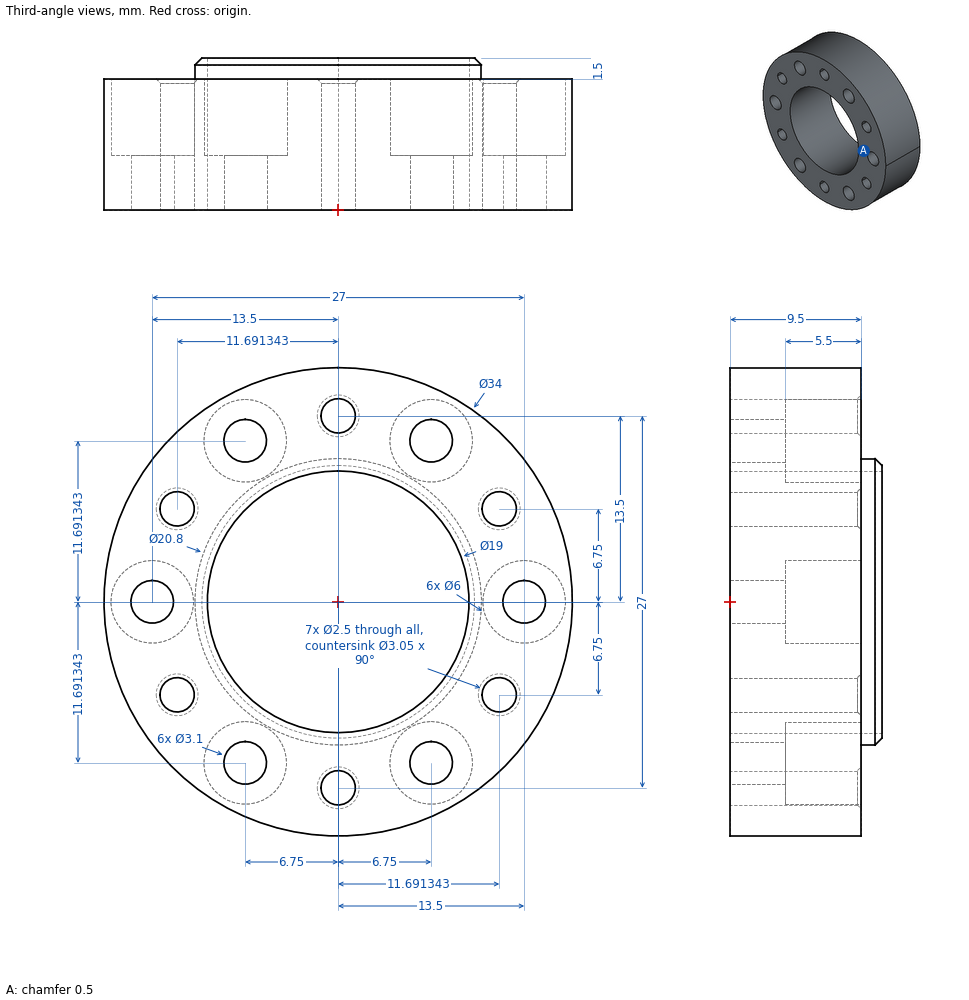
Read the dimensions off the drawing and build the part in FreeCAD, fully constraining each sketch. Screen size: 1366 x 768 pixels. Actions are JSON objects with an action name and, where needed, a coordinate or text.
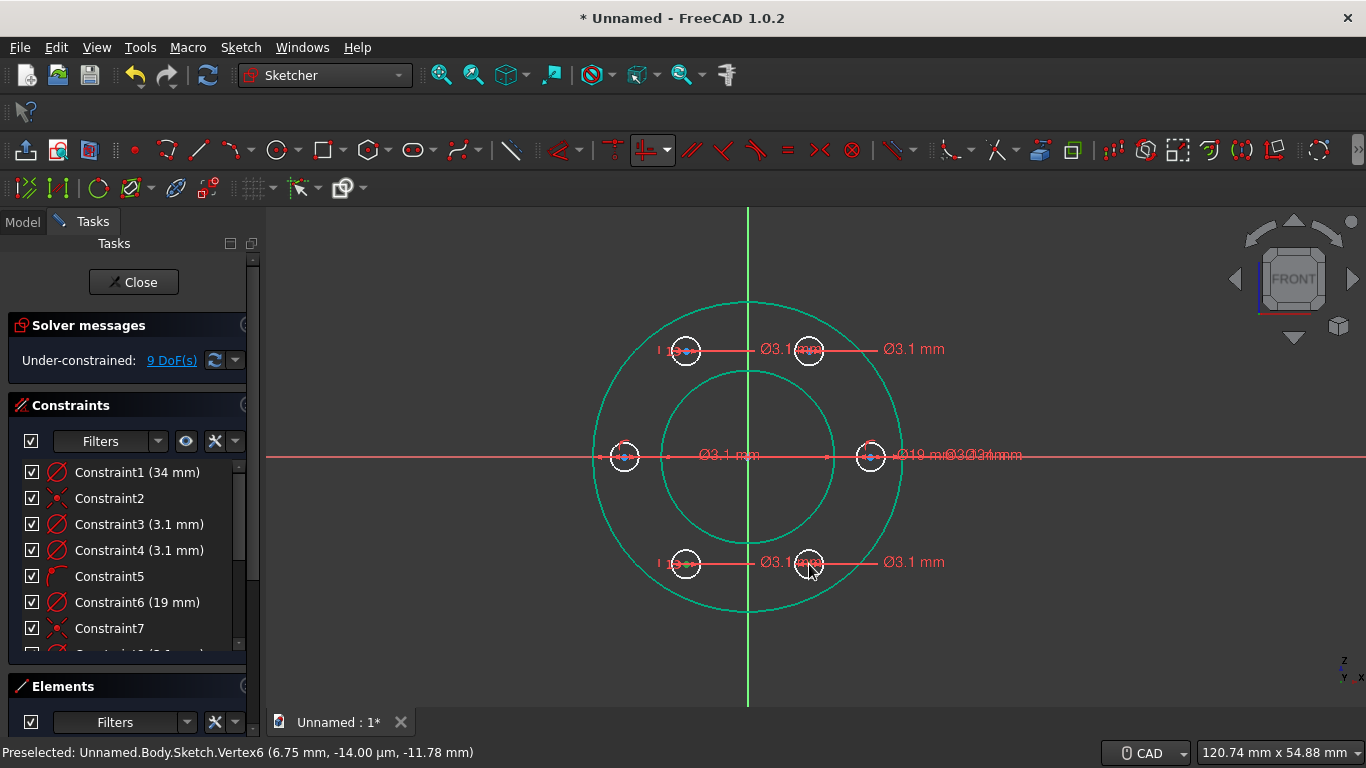
{"action": "left_click", "coordinate": [670, 150]}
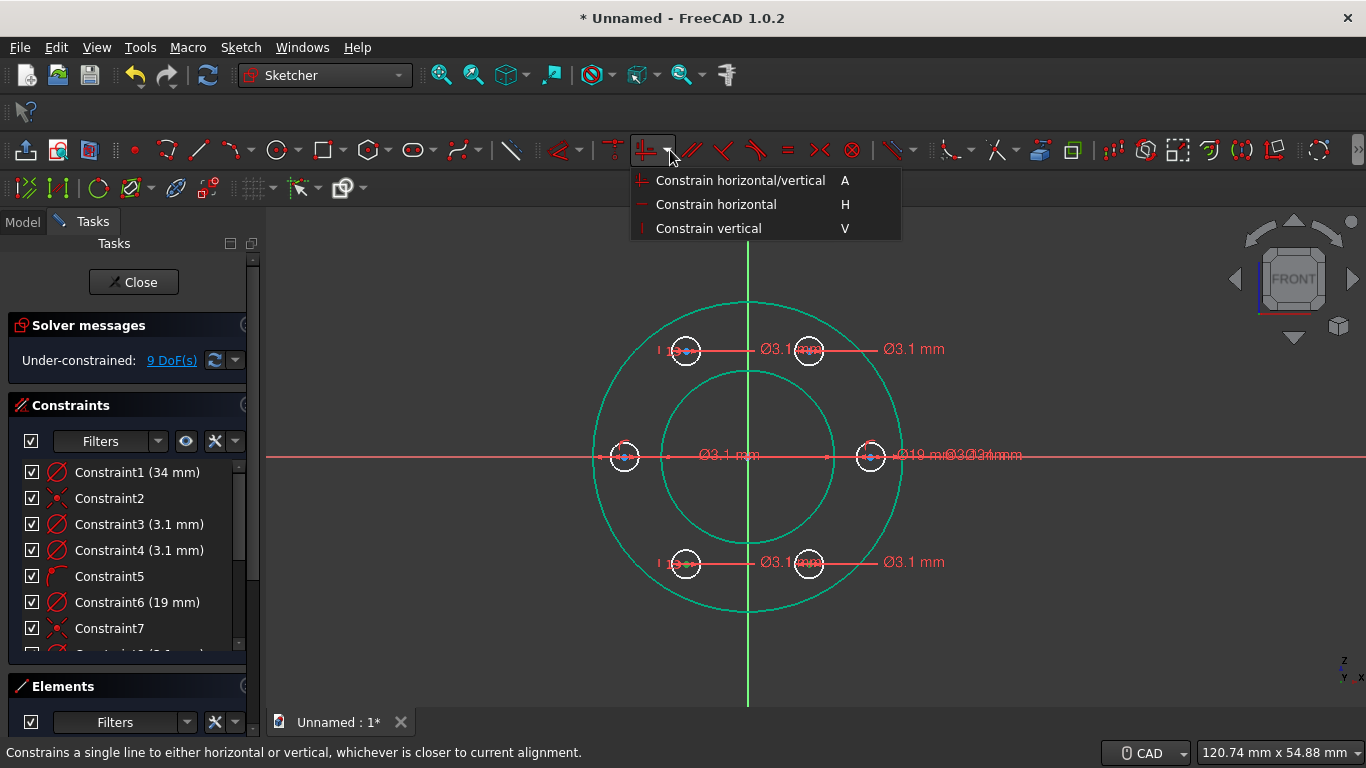
{"action": "left_click", "coordinate": [766, 204]}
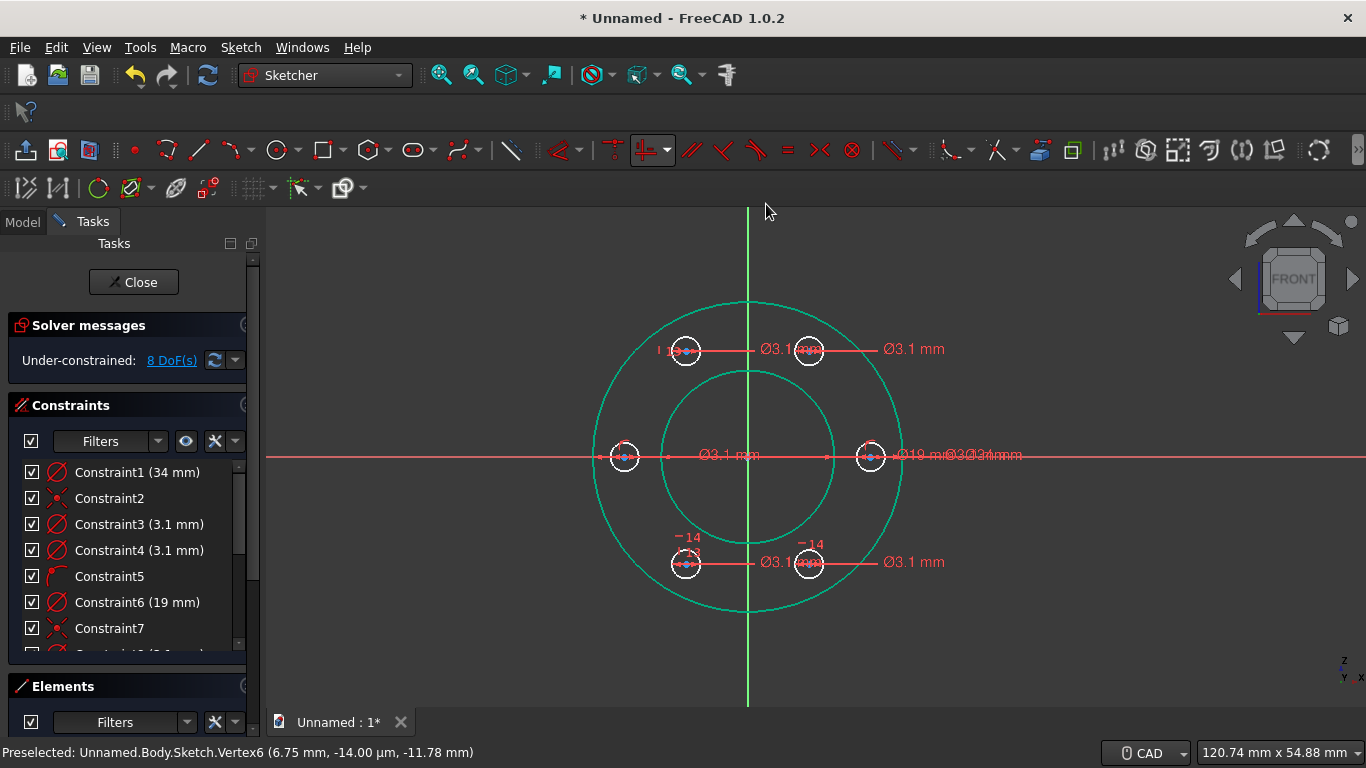
{"action": "left_click", "coordinate": [809, 564]}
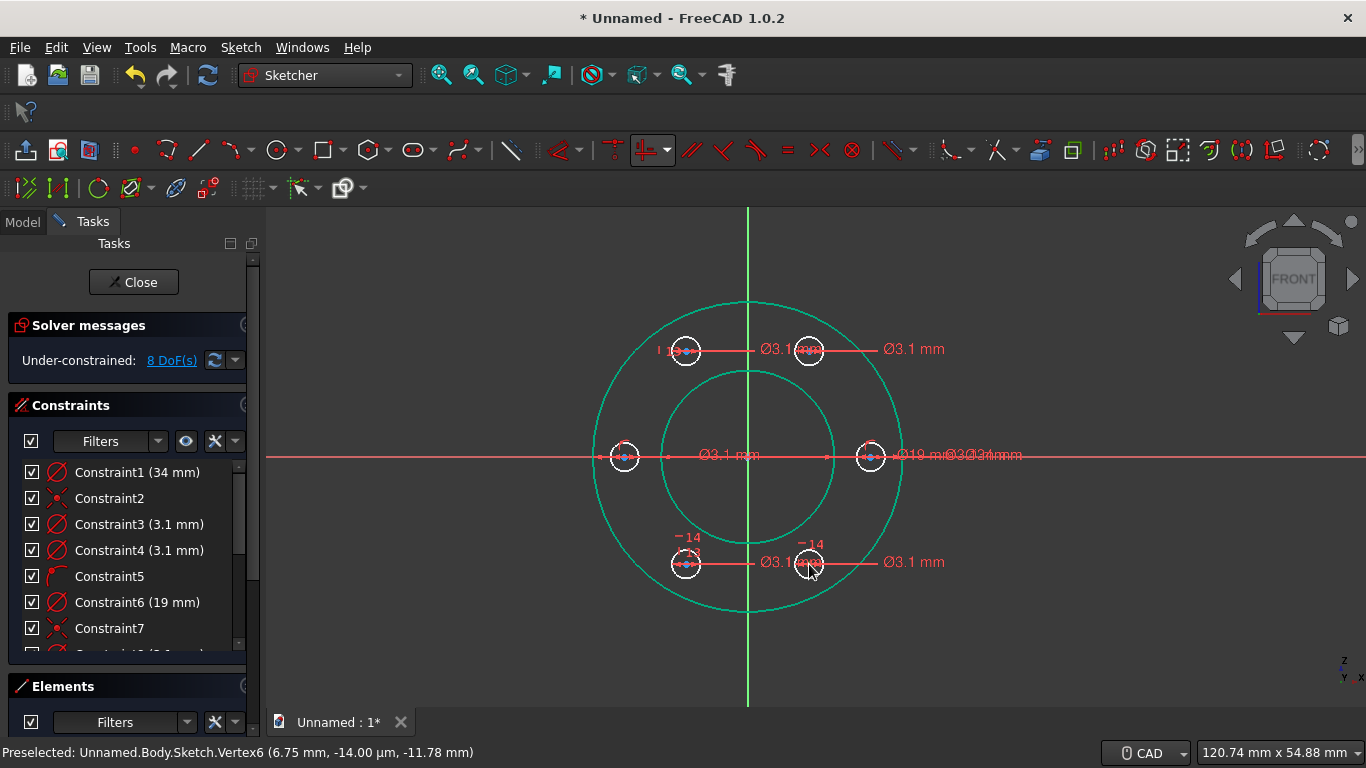
{"action": "left_click", "coordinate": [809, 351]}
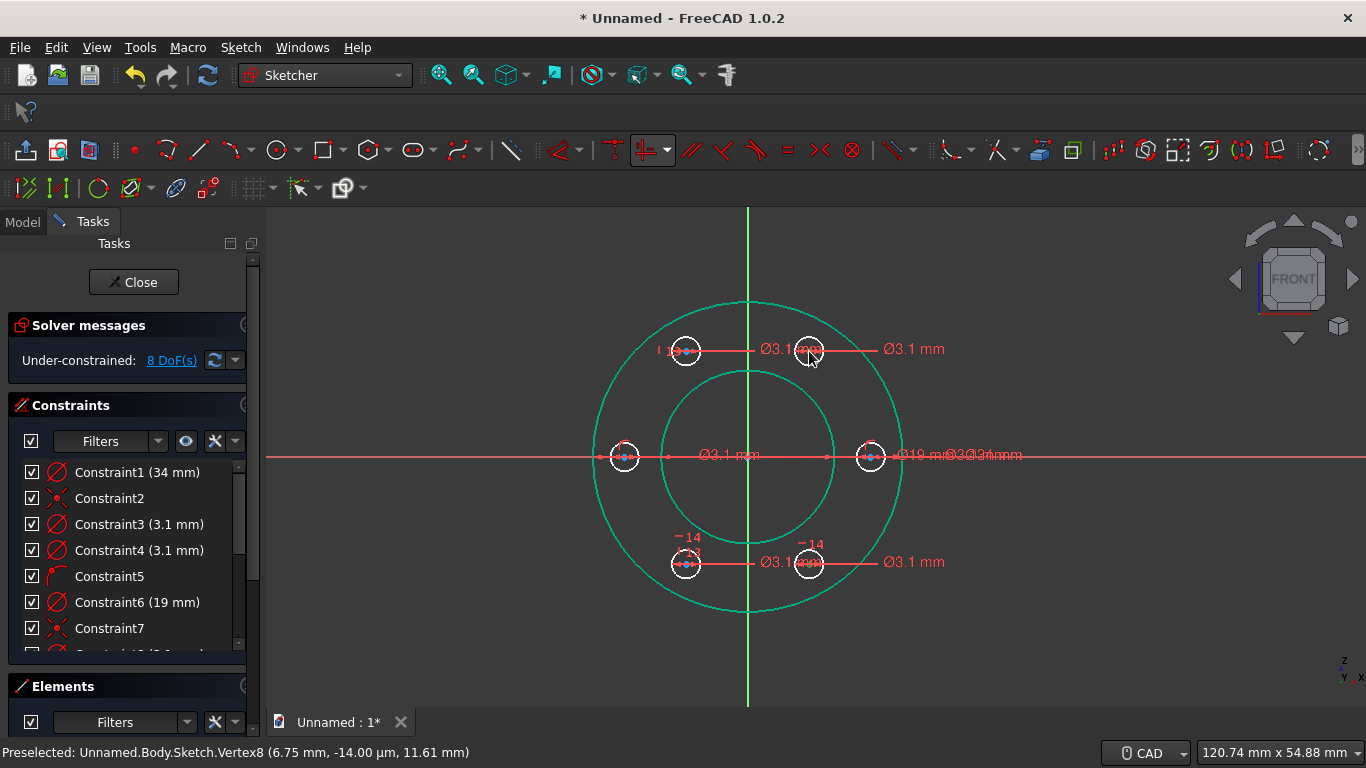
{"action": "key", "text": "v"}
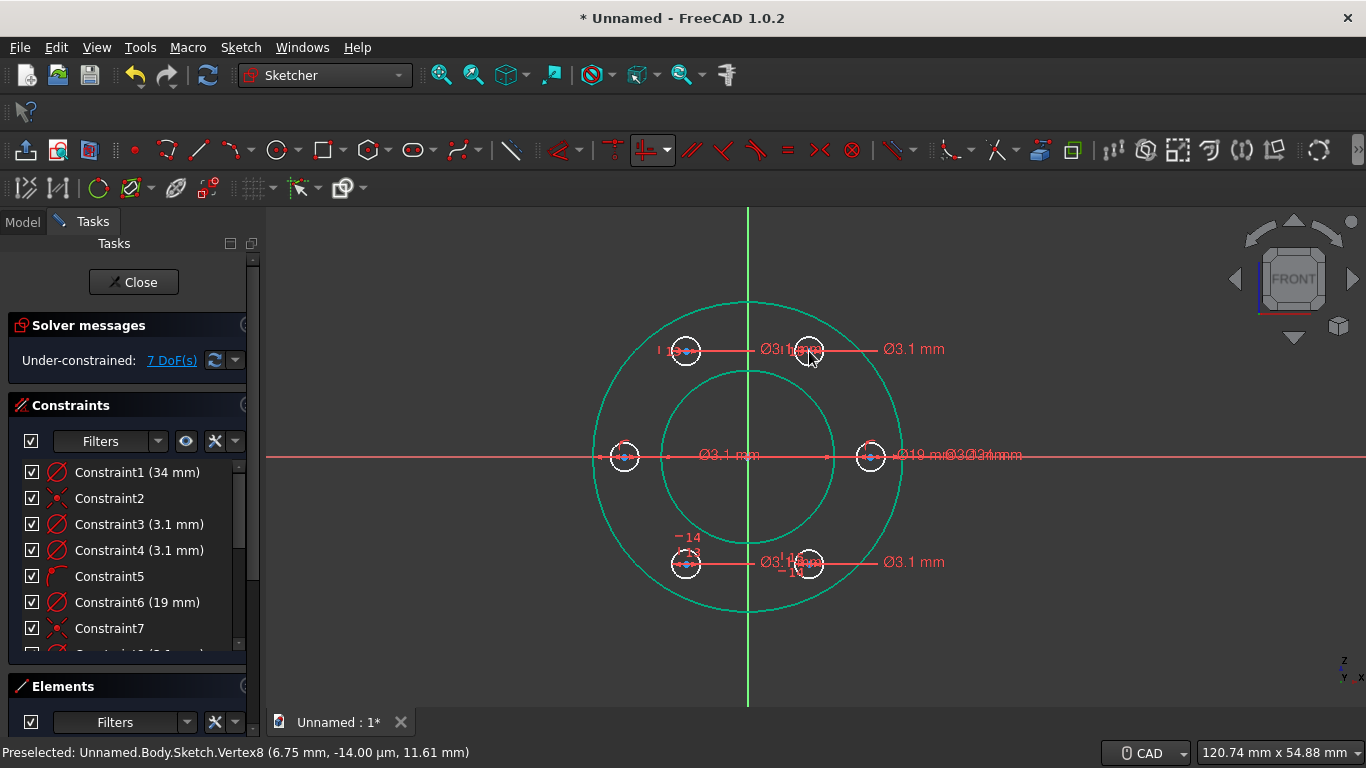
{"action": "left_click", "coordinate": [686, 351]}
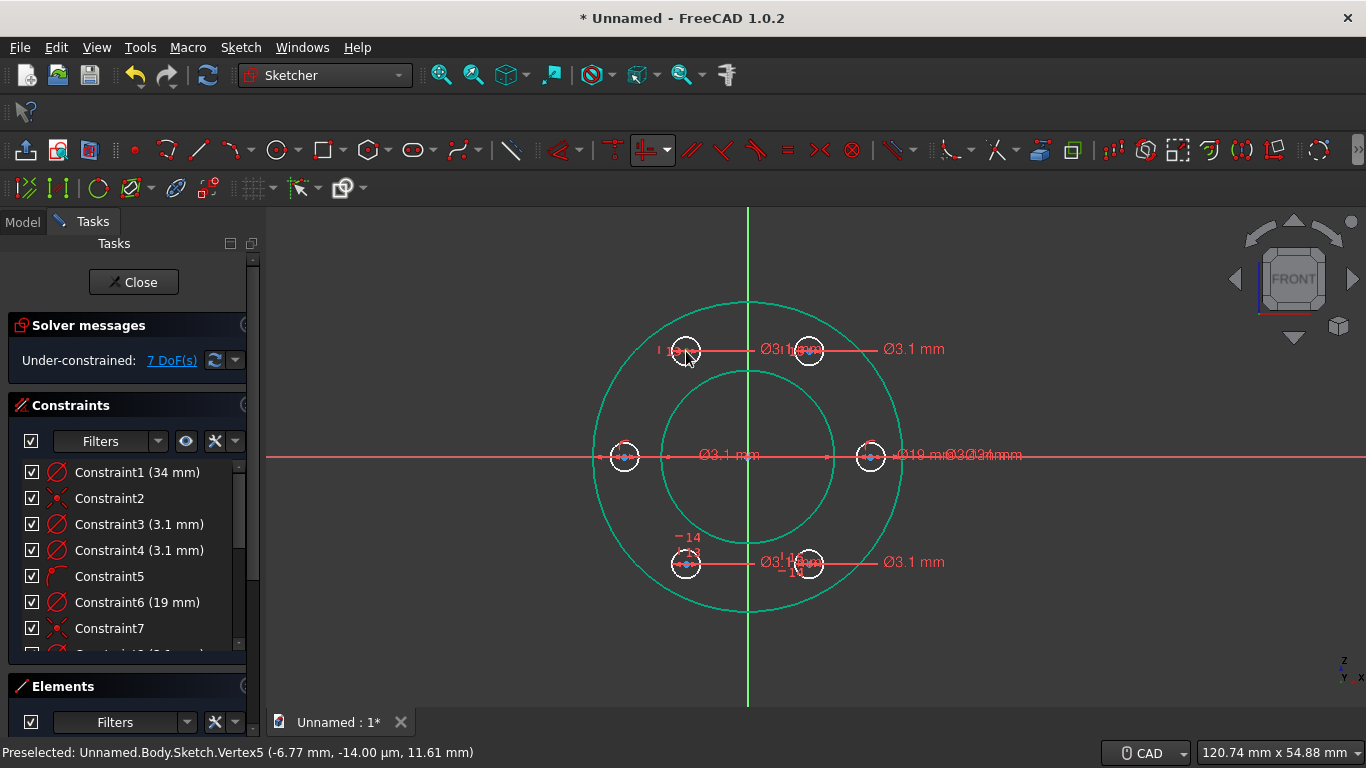
{"action": "left_click", "coordinate": [809, 351]}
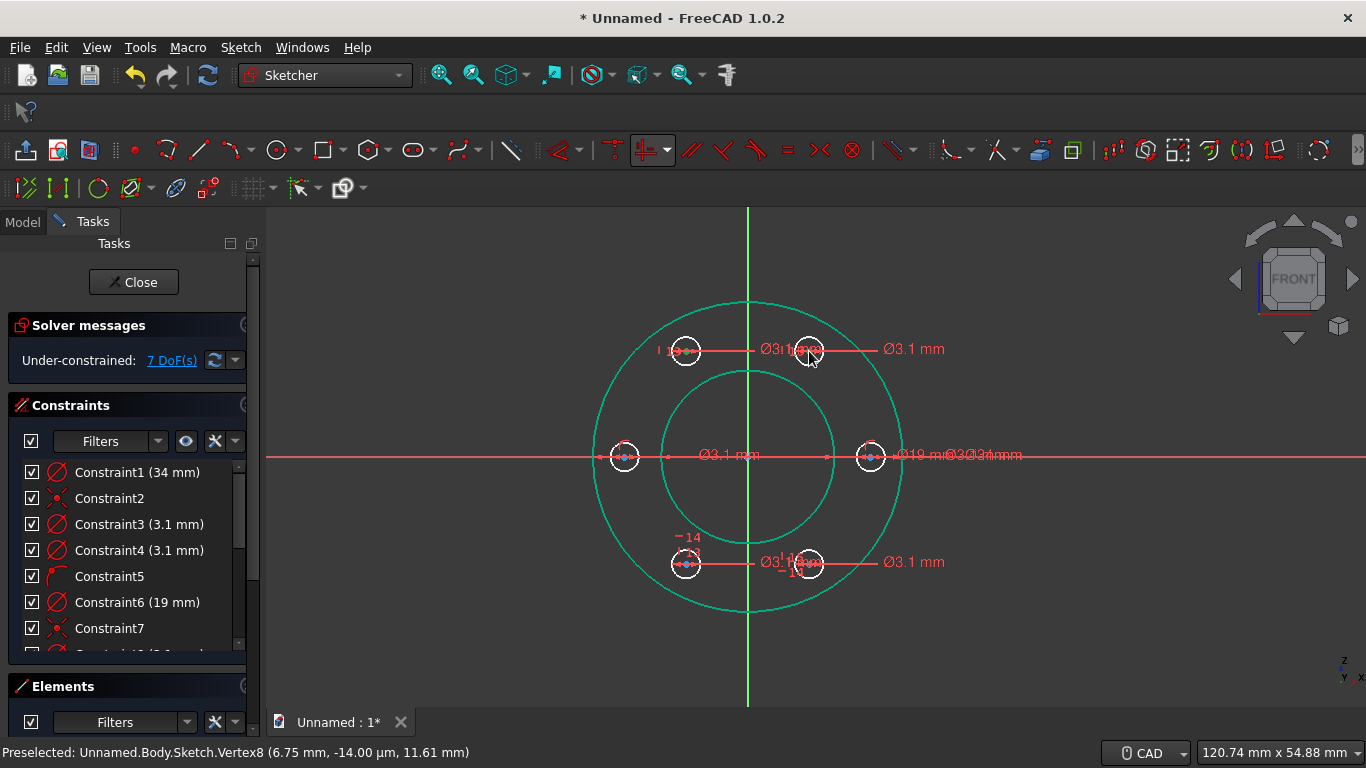
{"action": "left_click", "coordinate": [670, 150]}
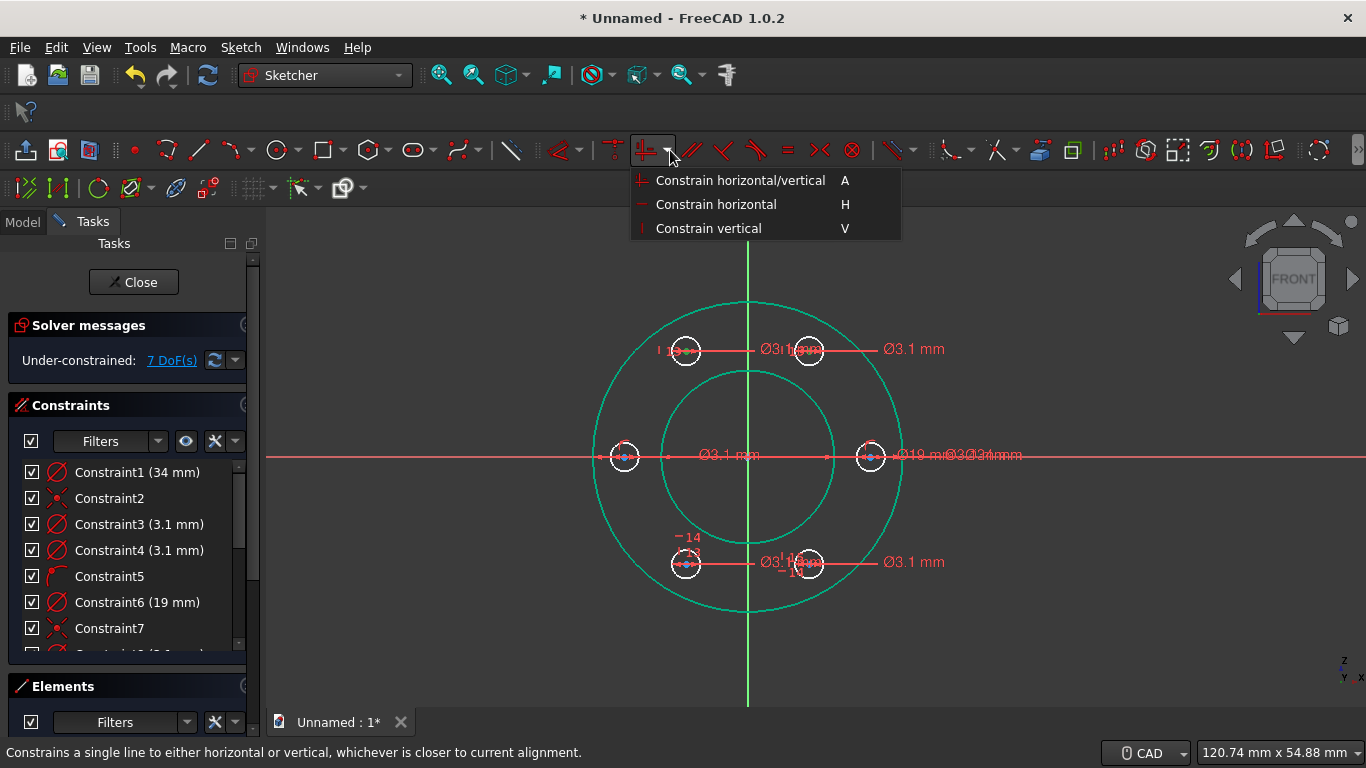
{"action": "left_click", "coordinate": [766, 204]}